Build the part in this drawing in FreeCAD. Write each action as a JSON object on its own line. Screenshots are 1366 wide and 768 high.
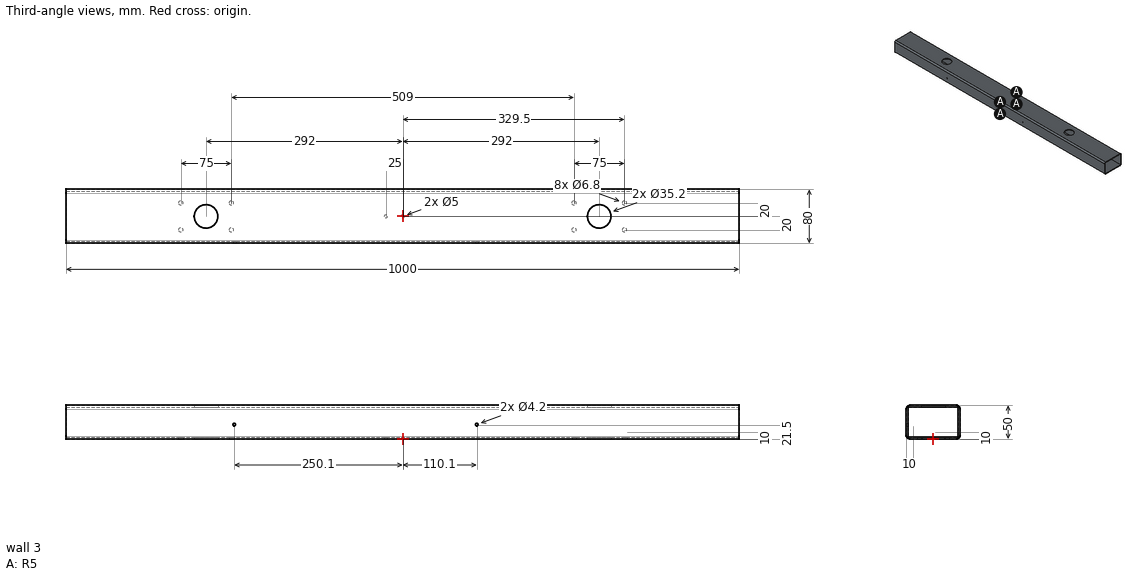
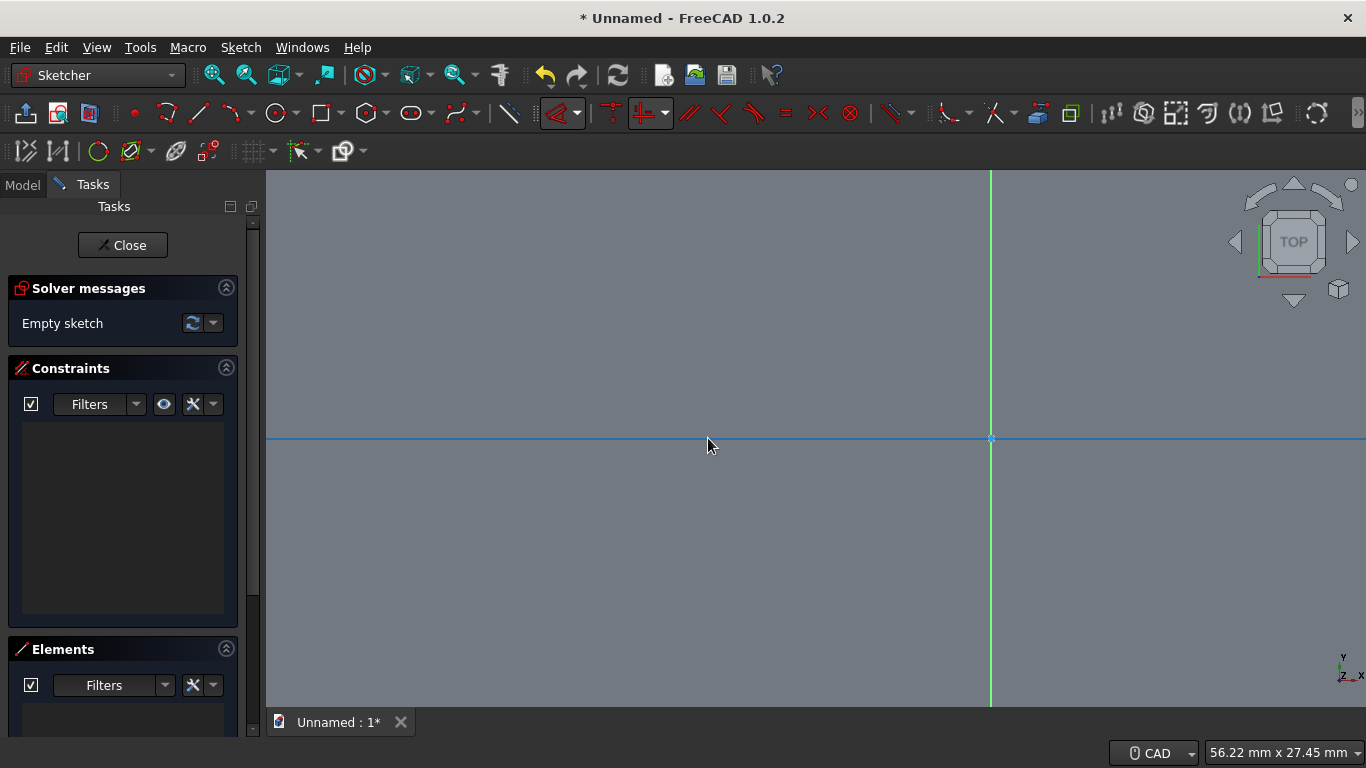
{"action": "left_click", "coordinate": [276, 114]}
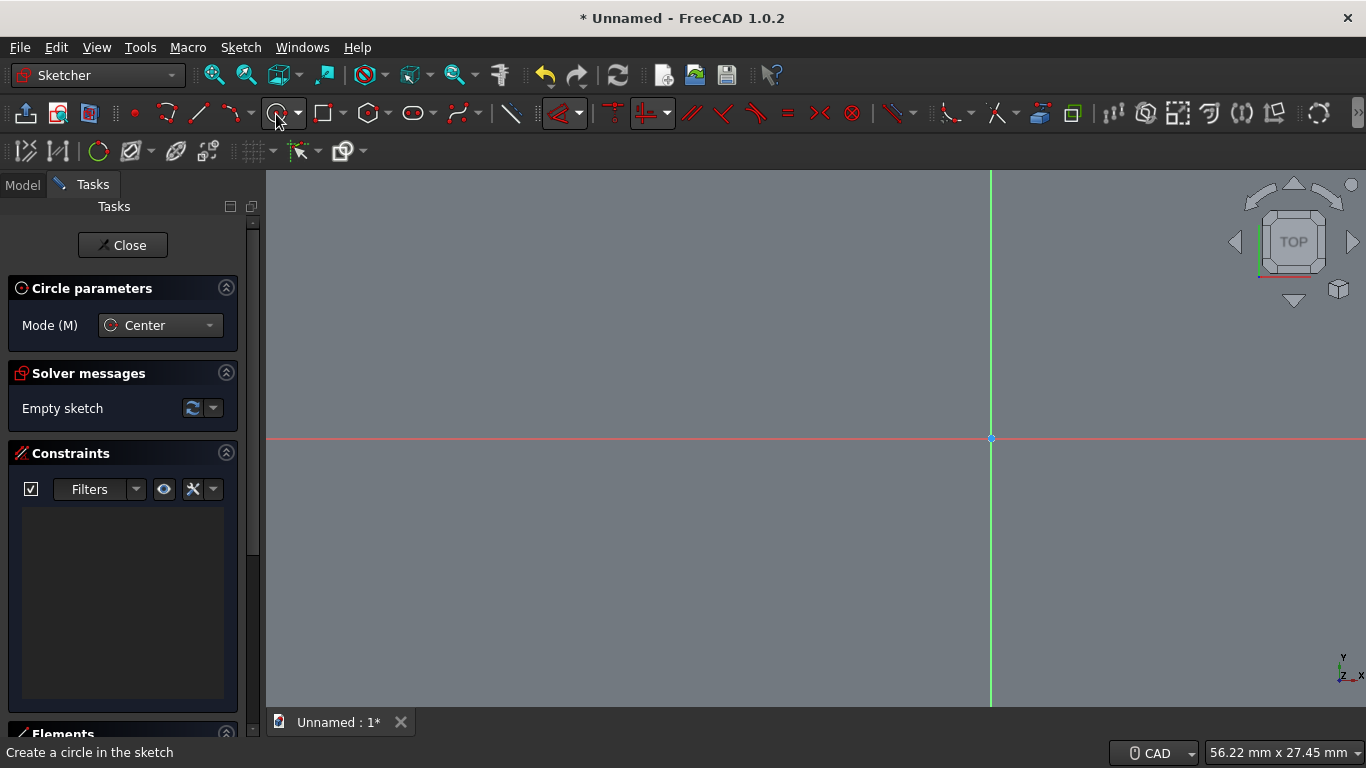
{"action": "left_click", "coordinate": [991, 438]}
{"action": "mouse_move", "coordinate": [1026, 404]}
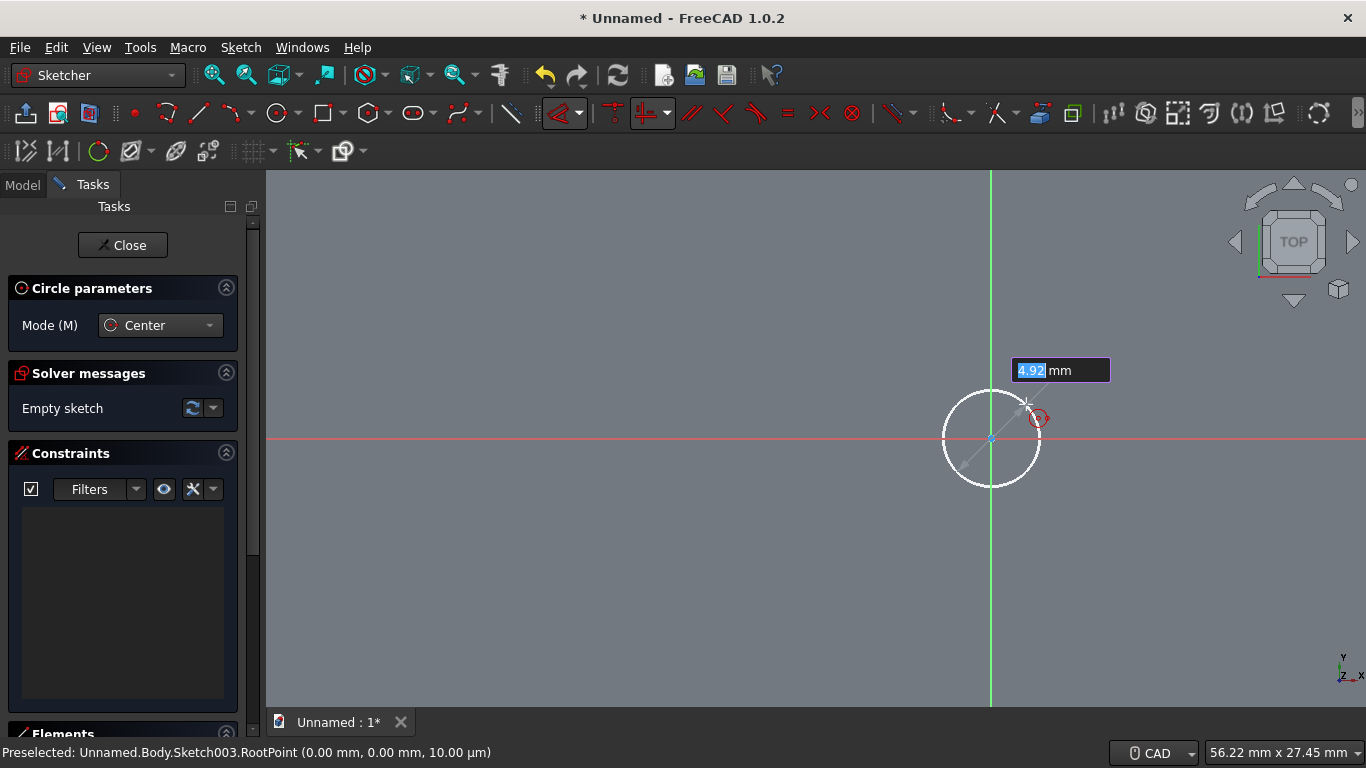
{"action": "type", "text": "5"}
{"action": "key", "text": "Return"}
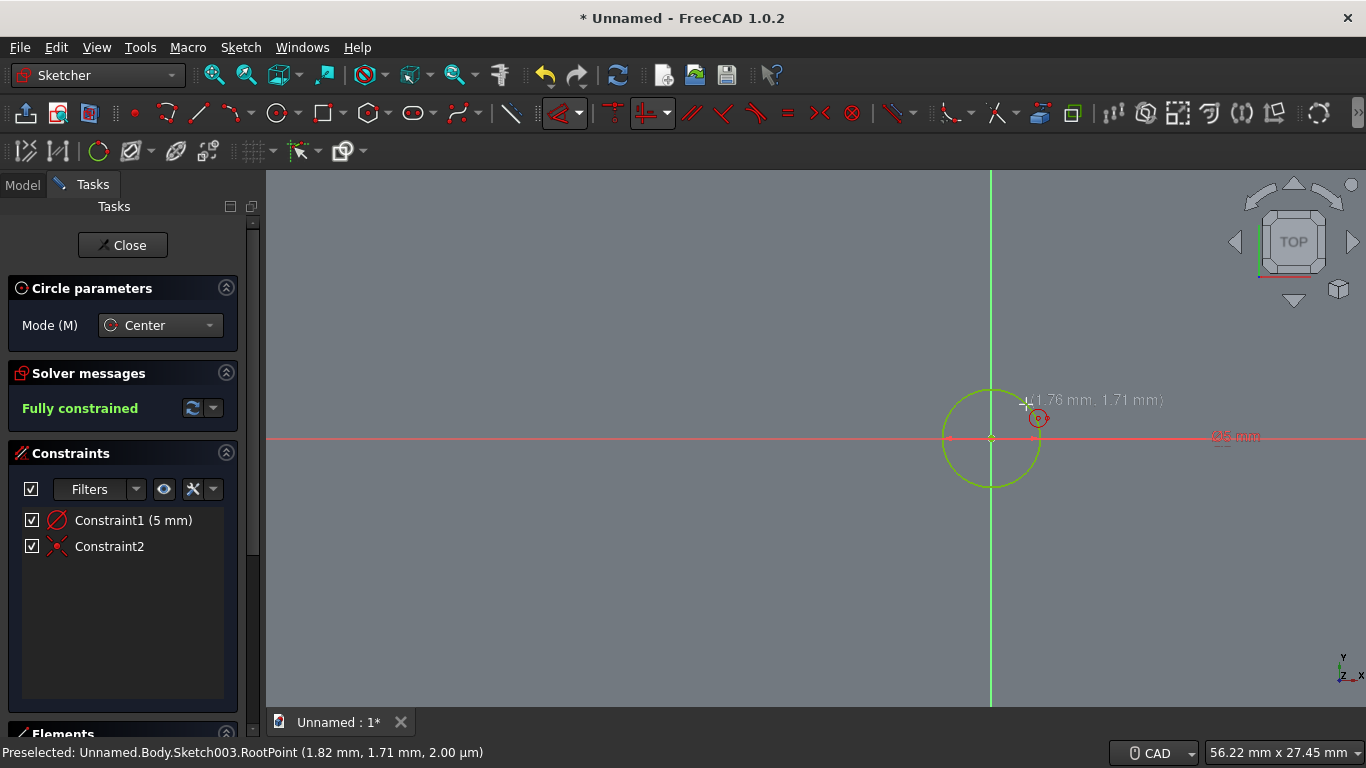
{"action": "left_click", "coordinate": [502, 438]}
{"action": "mouse_move", "coordinate": [537, 404]}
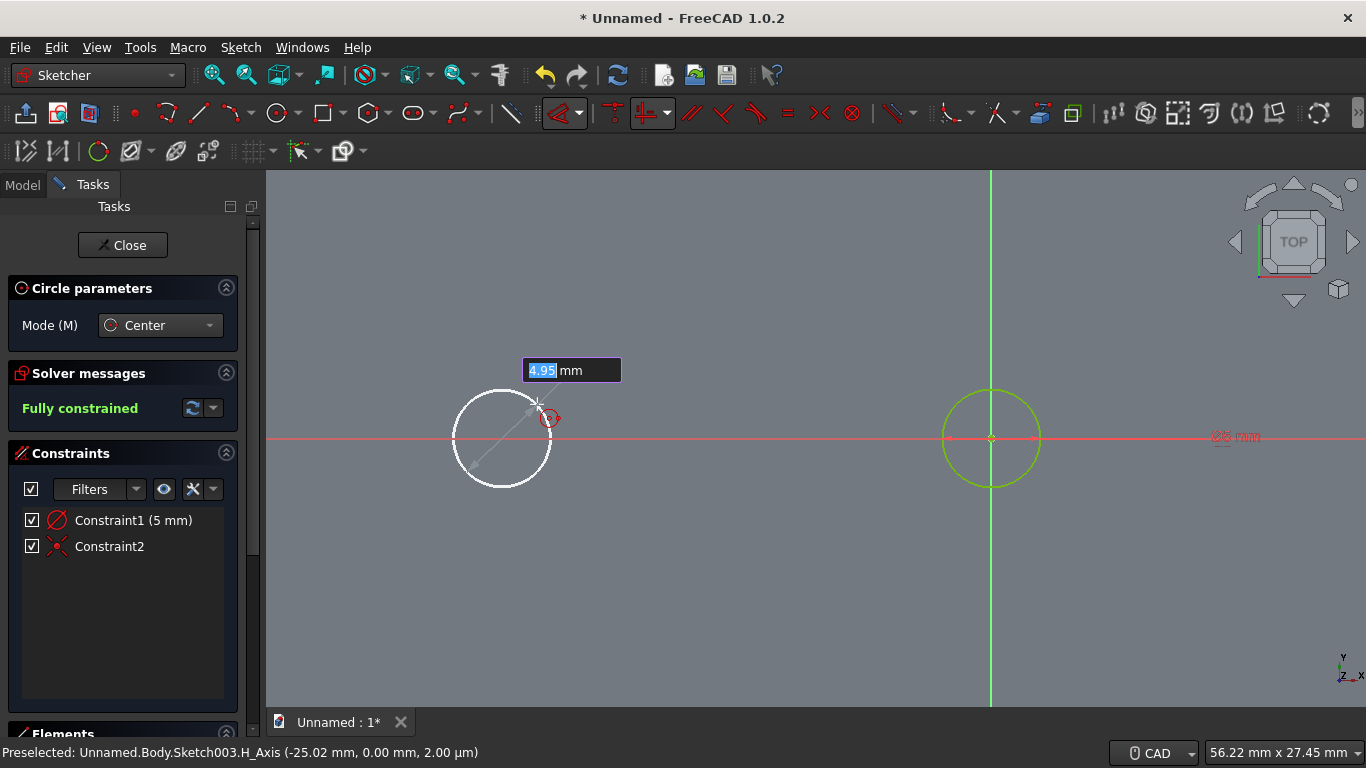
{"action": "type", "text": "5"}
{"action": "key", "text": "Return"}
{"action": "key", "text": "Escape"}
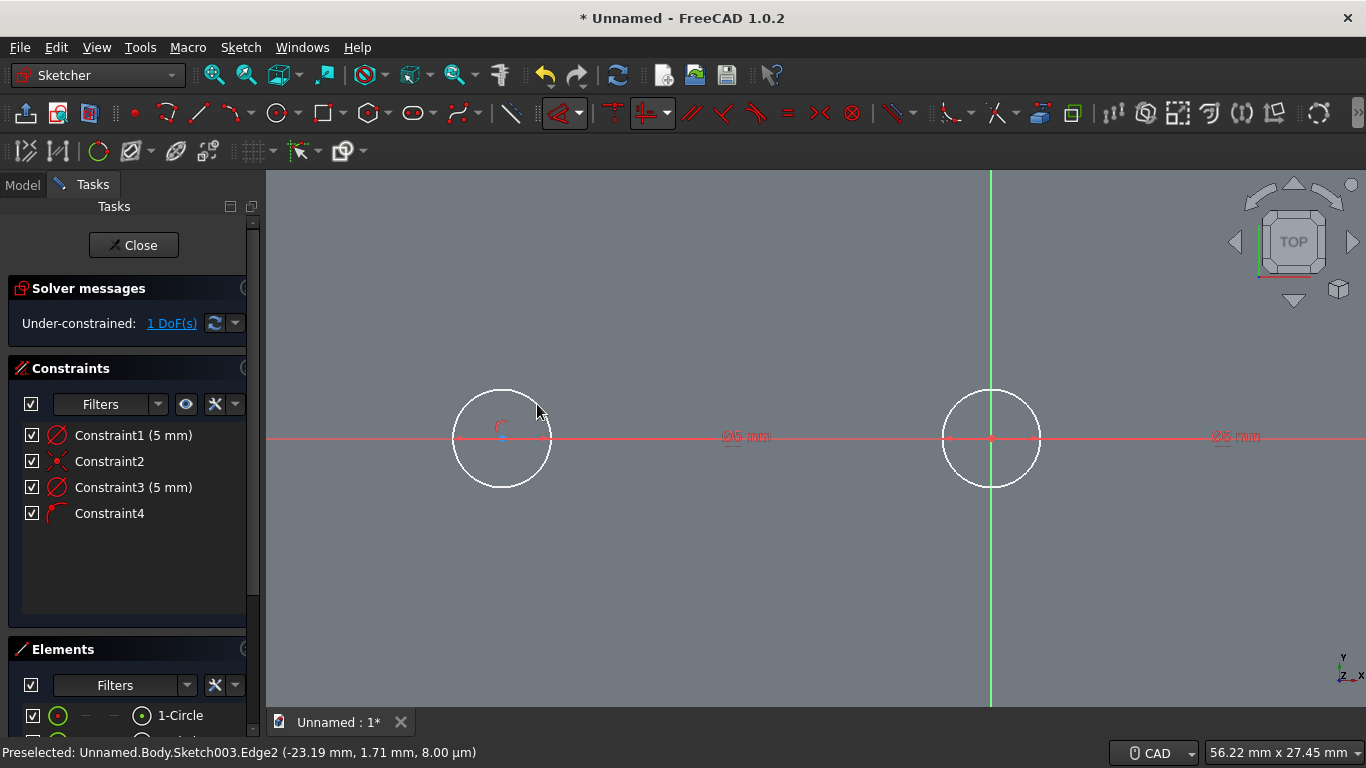
{"action": "left_click", "coordinate": [502, 438]}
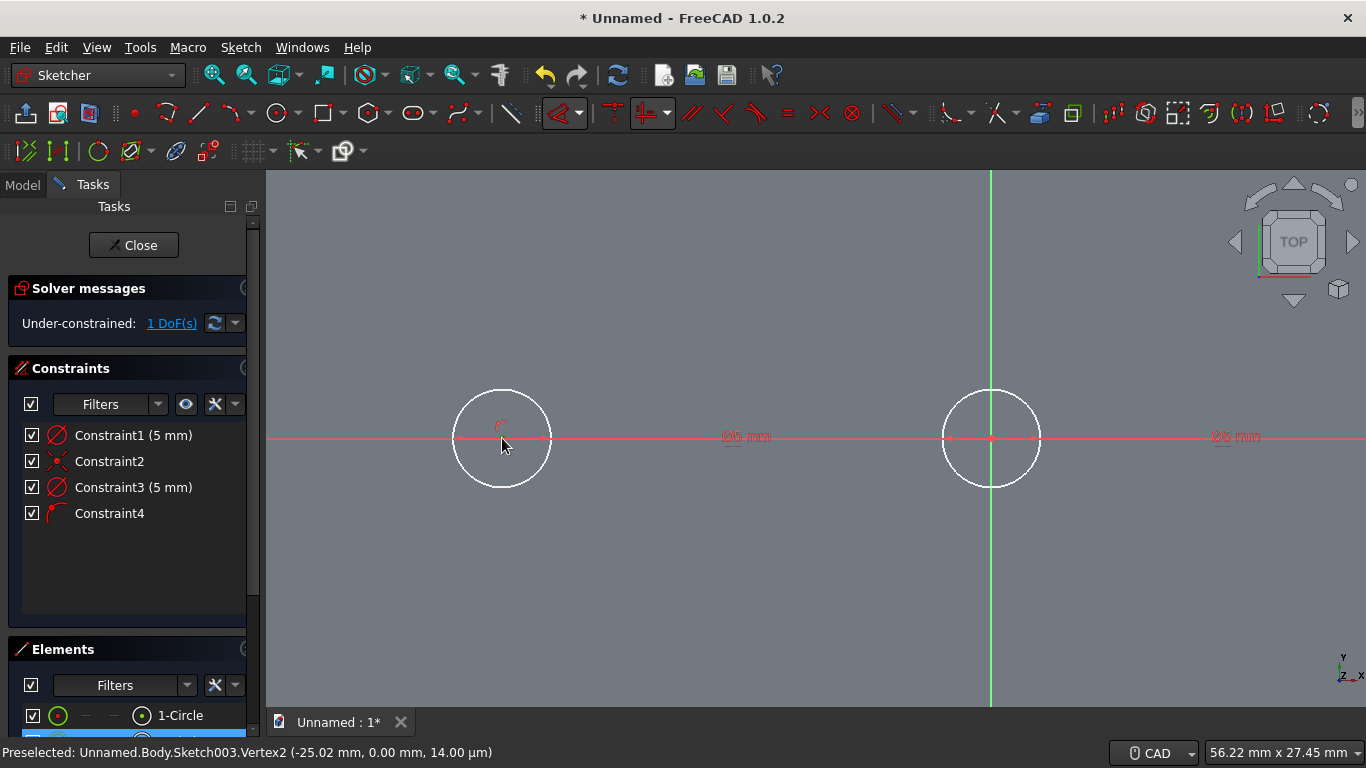
{"action": "key", "text": "l"}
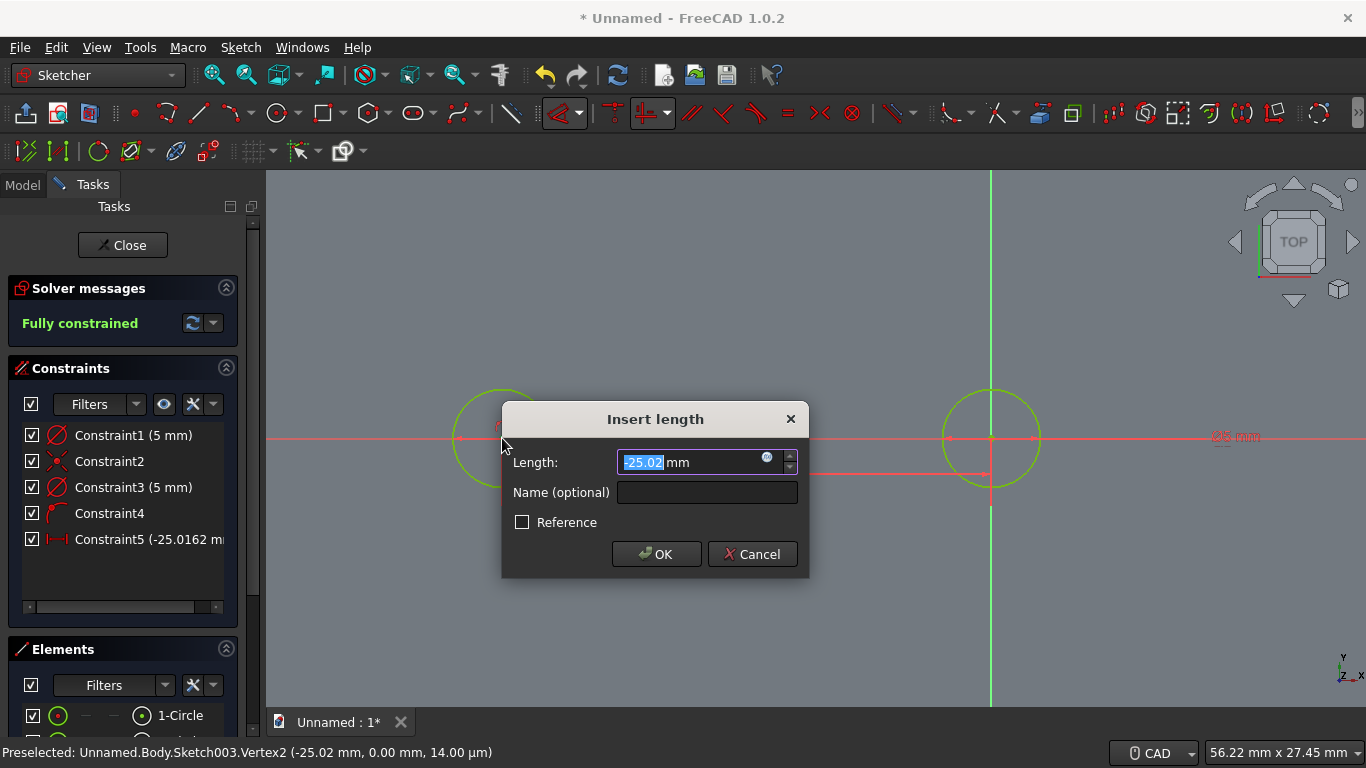
{"action": "type", "text": "-25"}
{"action": "key", "text": "Return"}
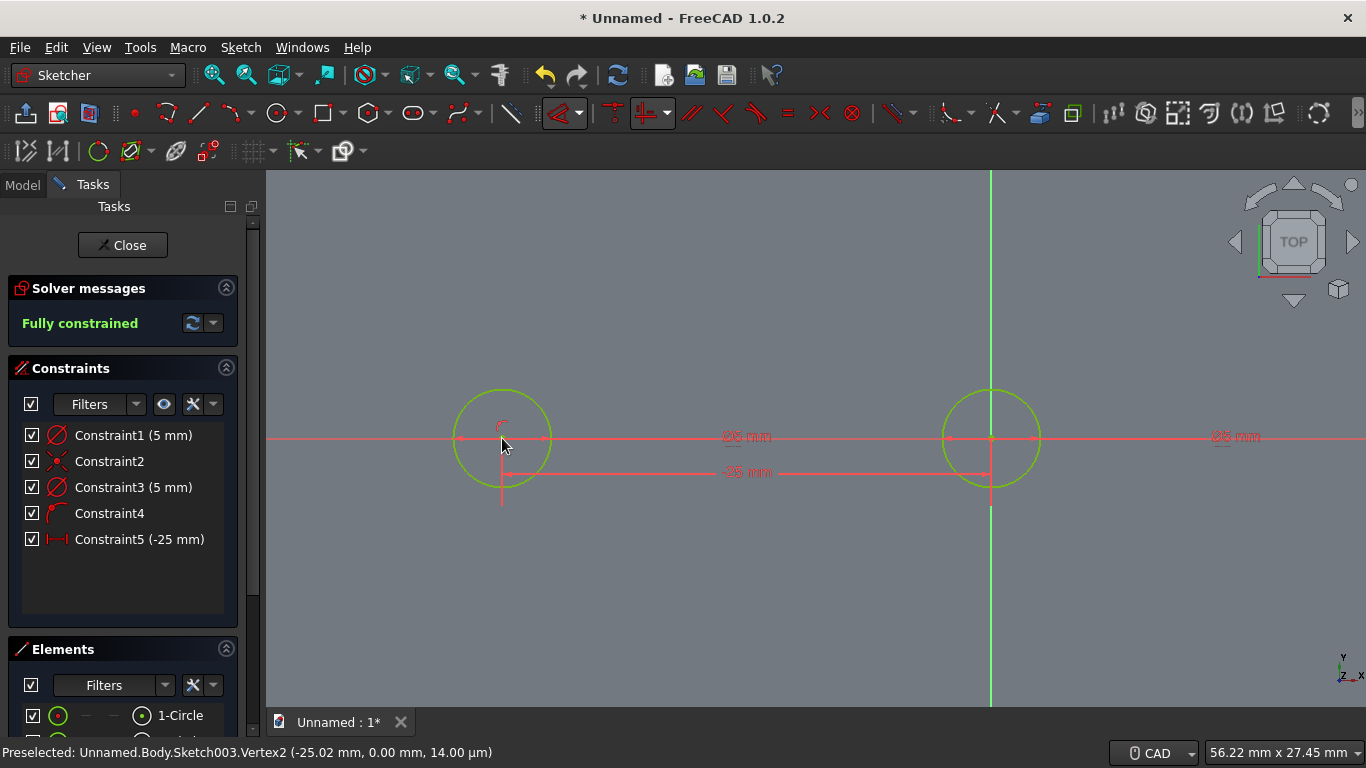
{"action": "left_click", "coordinate": [123, 245]}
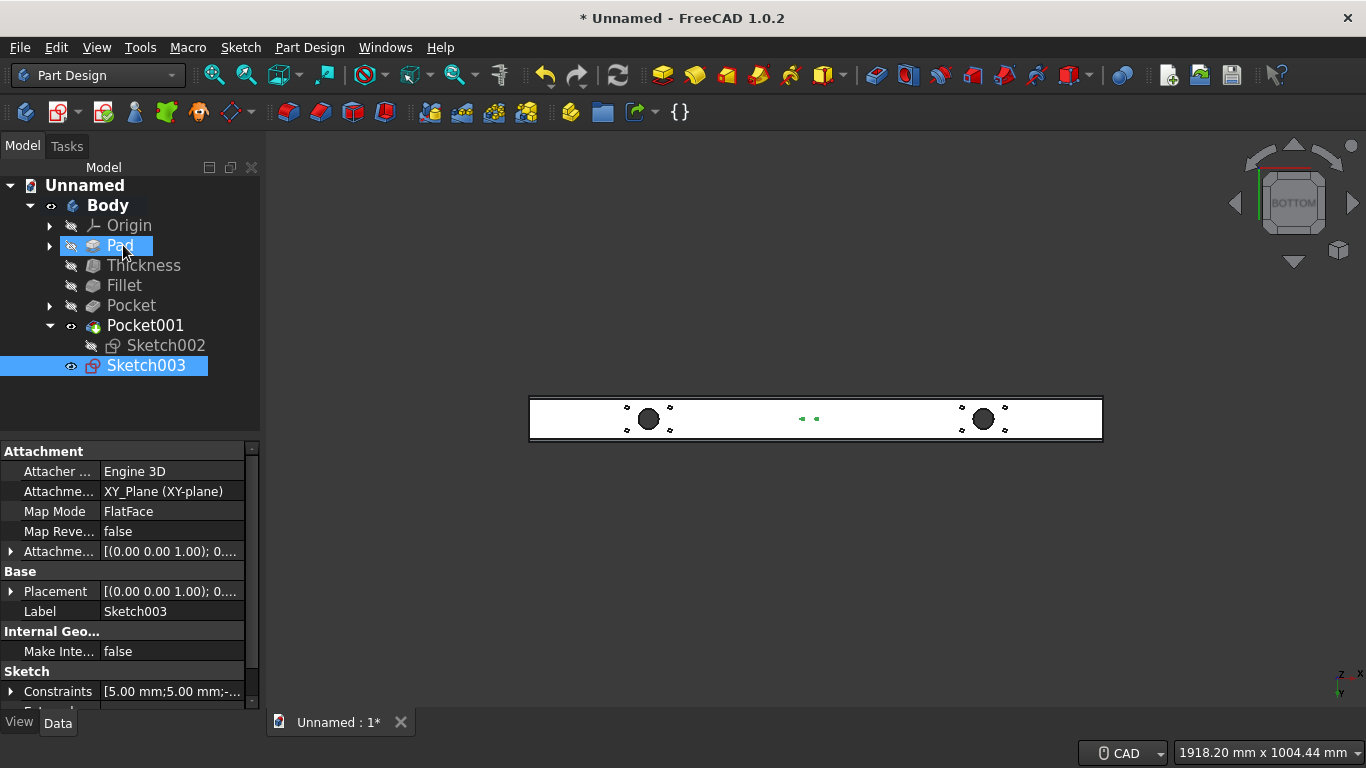
{"action": "left_click", "coordinate": [878, 76]}